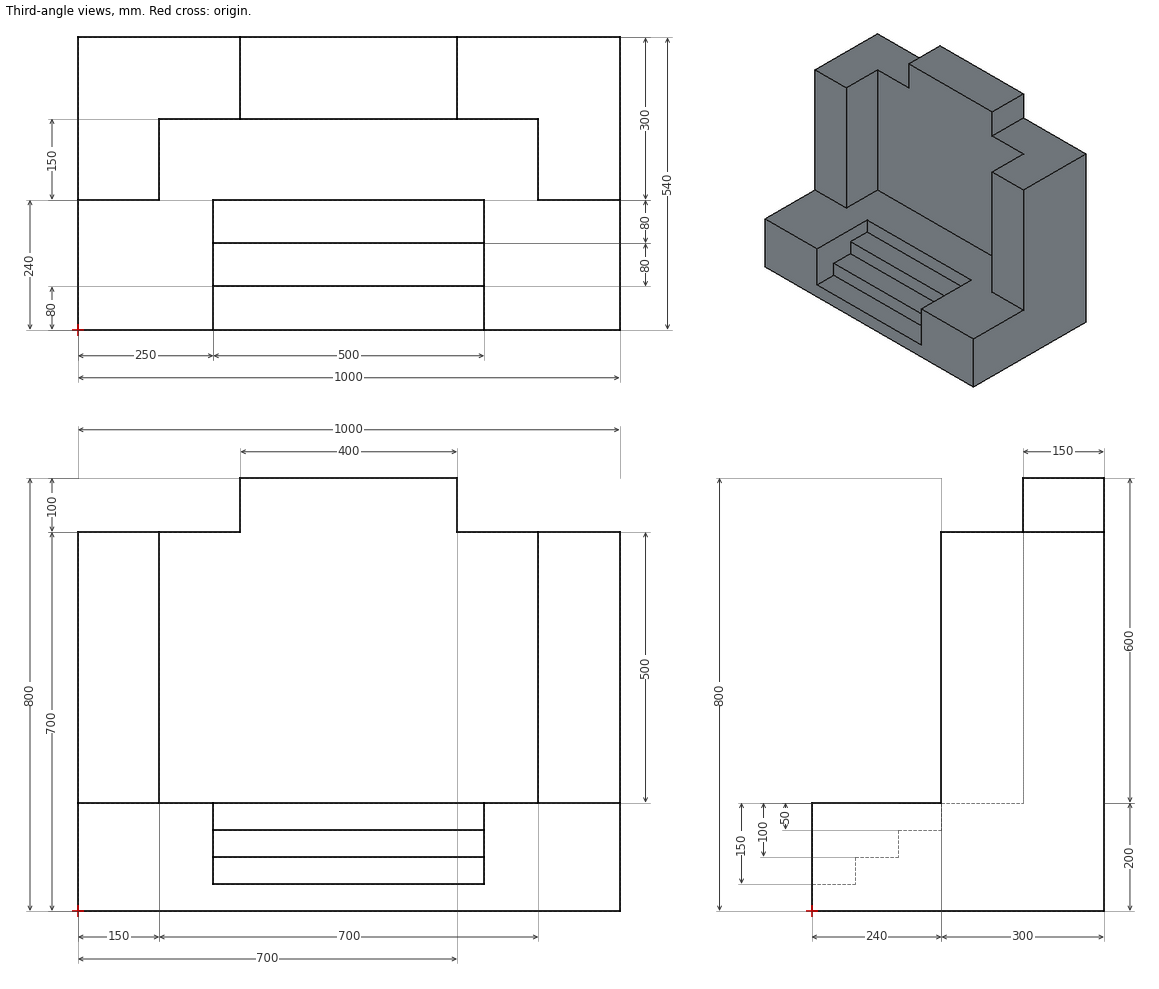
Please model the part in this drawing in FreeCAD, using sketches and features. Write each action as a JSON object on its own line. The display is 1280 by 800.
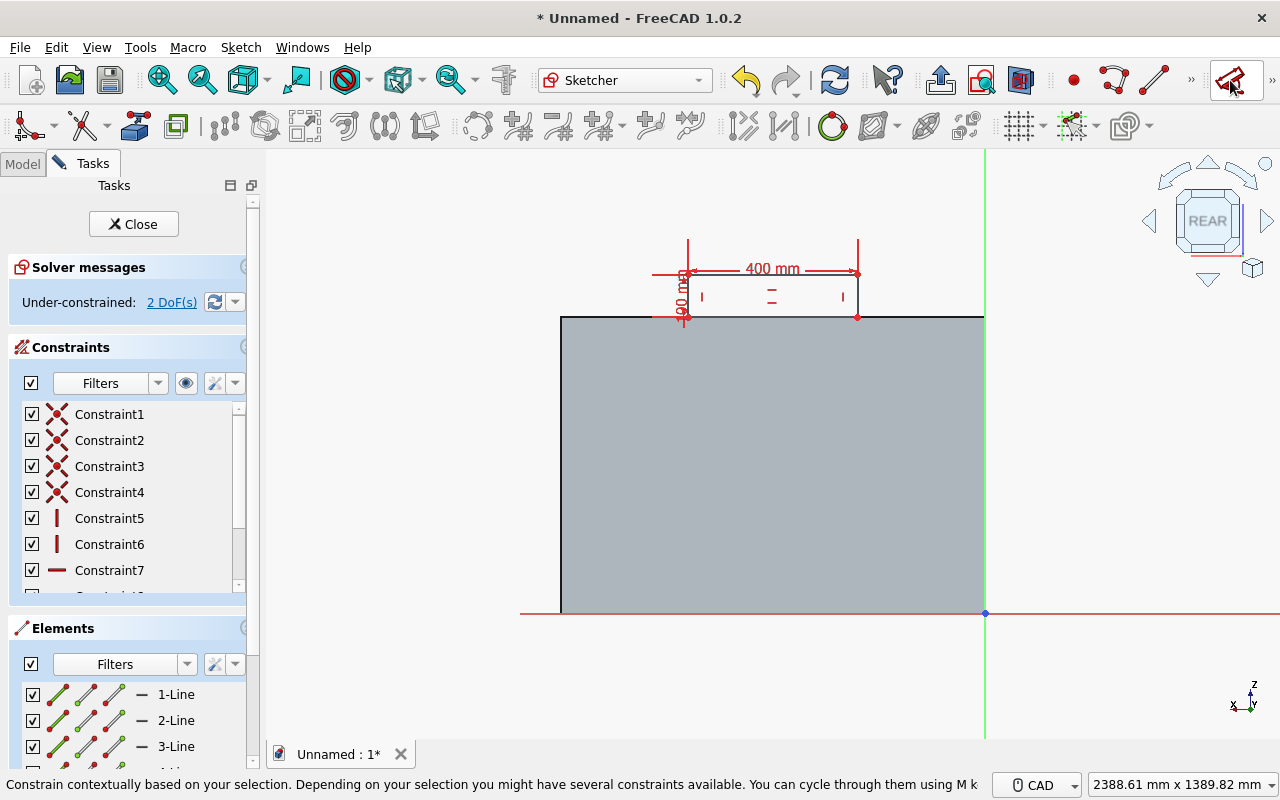
{"action": "left_click", "coordinate": [688, 275]}
{"action": "left_click", "coordinate": [837, 648]}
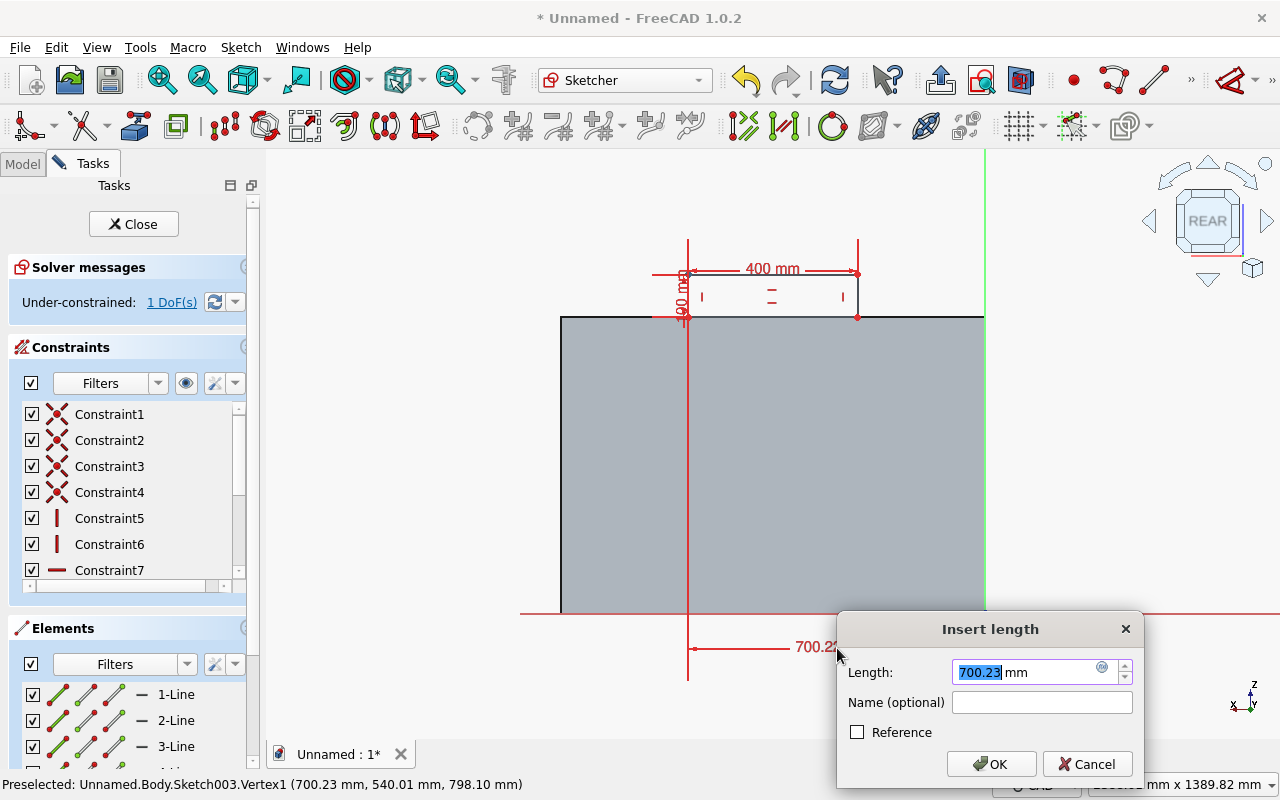
{"action": "type", "text": "700"}
{"action": "key", "text": "Return"}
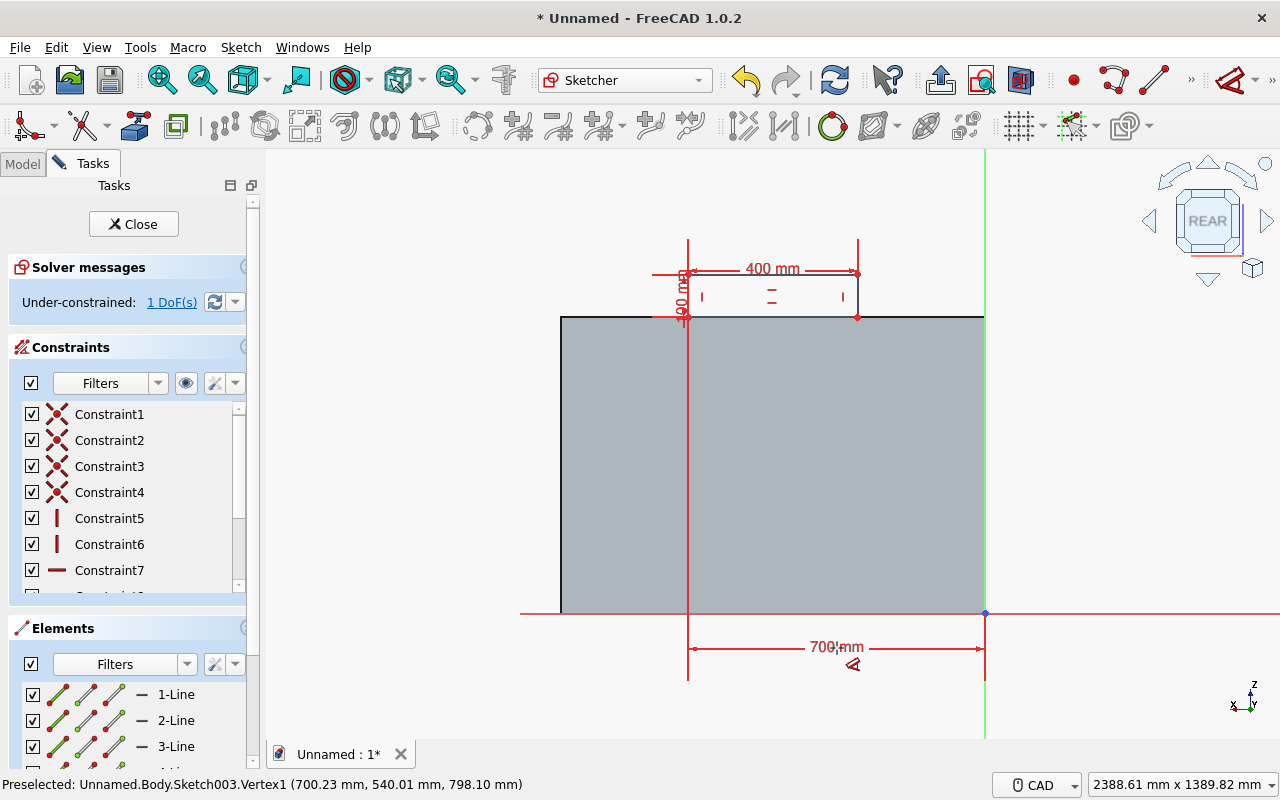
{"action": "left_click", "coordinate": [688, 275]}
{"action": "left_click", "coordinate": [1019, 444]}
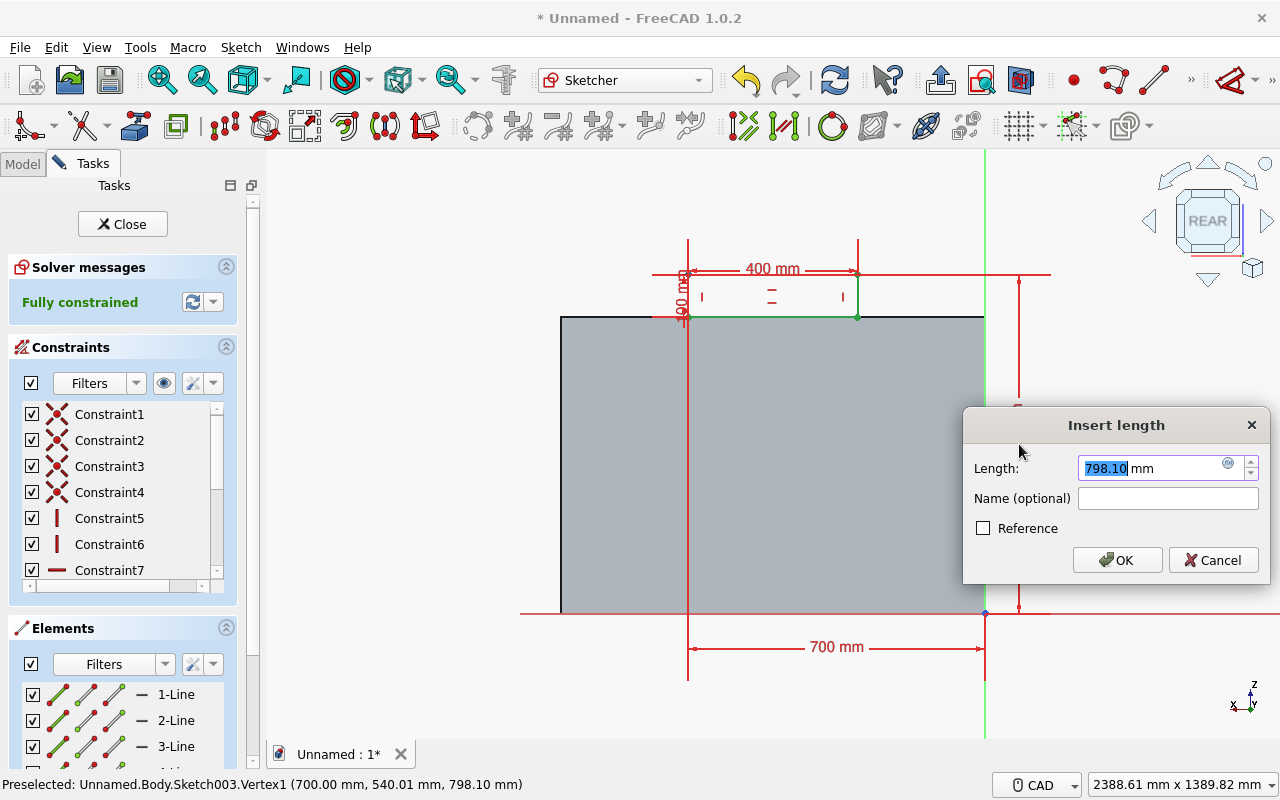
{"action": "type", "text": "800"}
{"action": "key", "text": "Return"}
{"action": "key", "text": "Escape"}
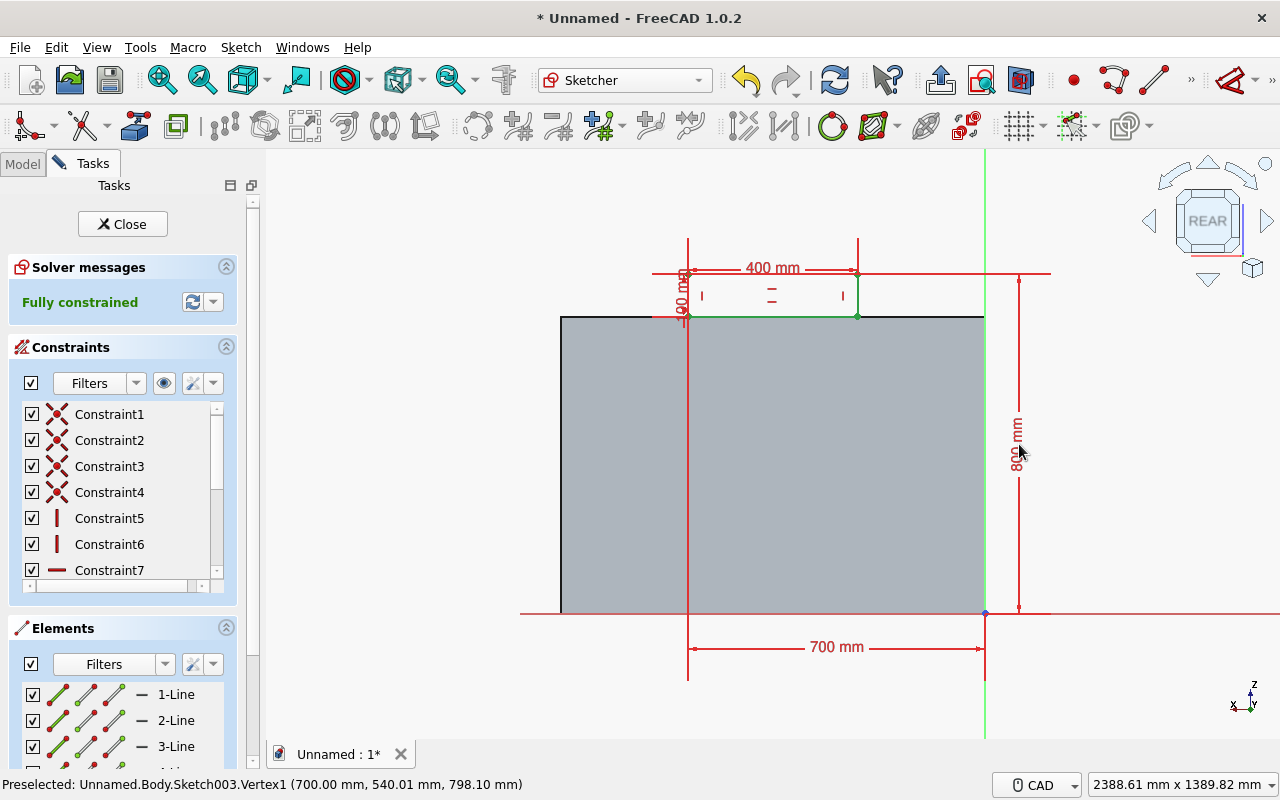
{"action": "left_click", "coordinate": [123, 224]}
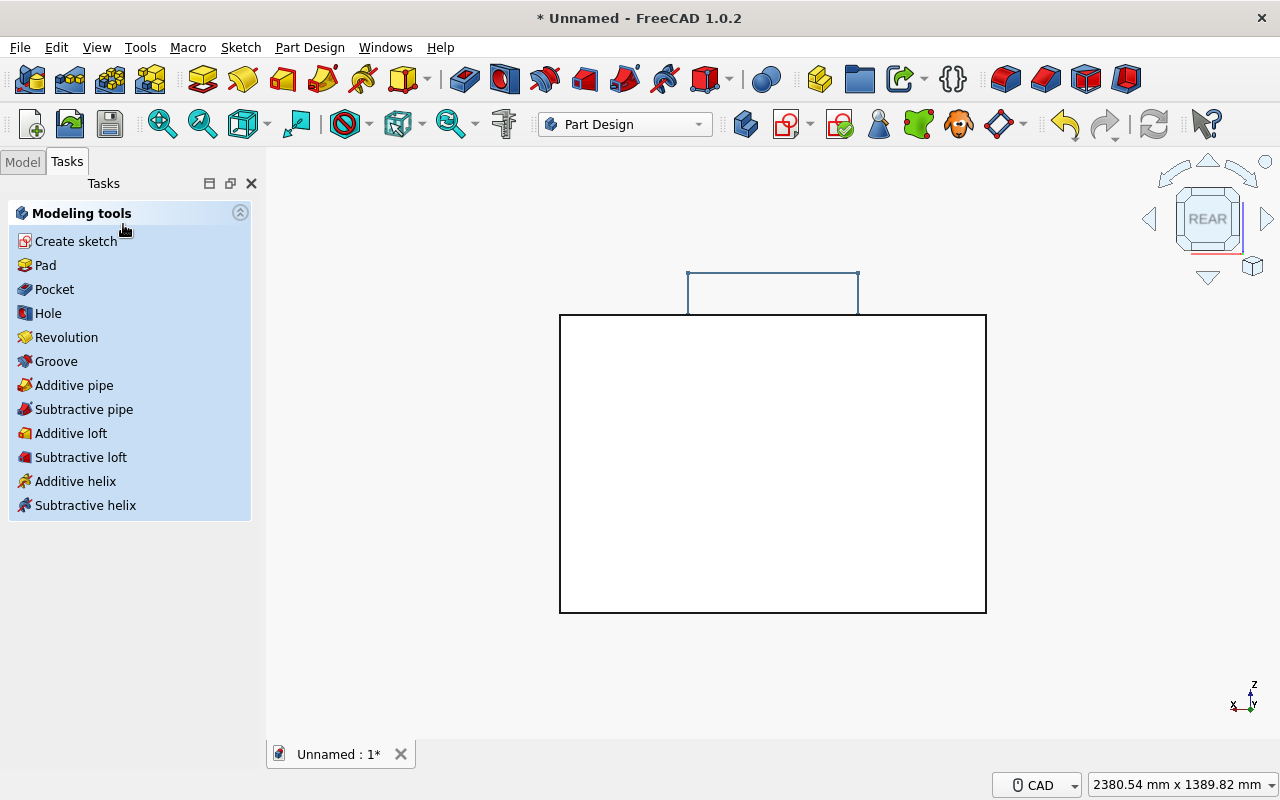
{"action": "left_click", "coordinate": [204, 80]}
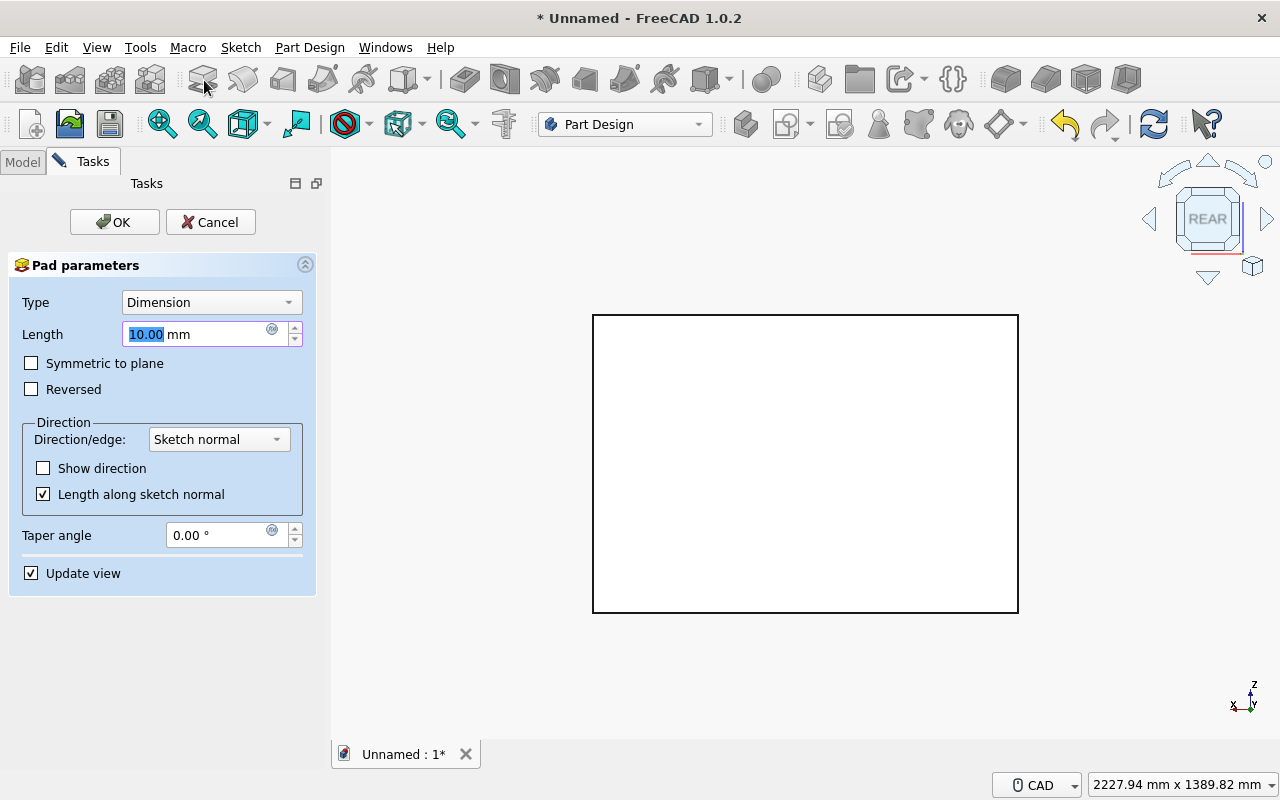
{"action": "type", "text": "150"}
{"action": "key", "text": "Tab"}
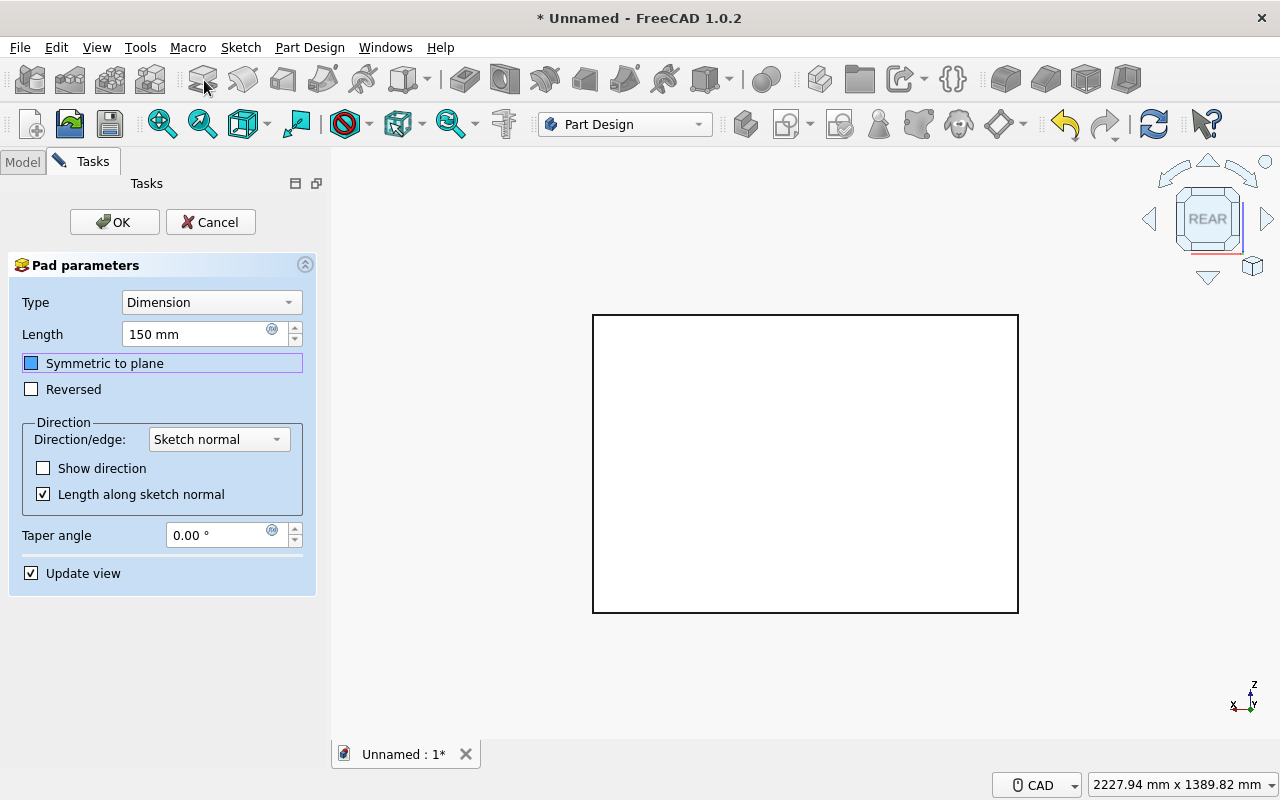
{"action": "left_click", "coordinate": [30, 389]}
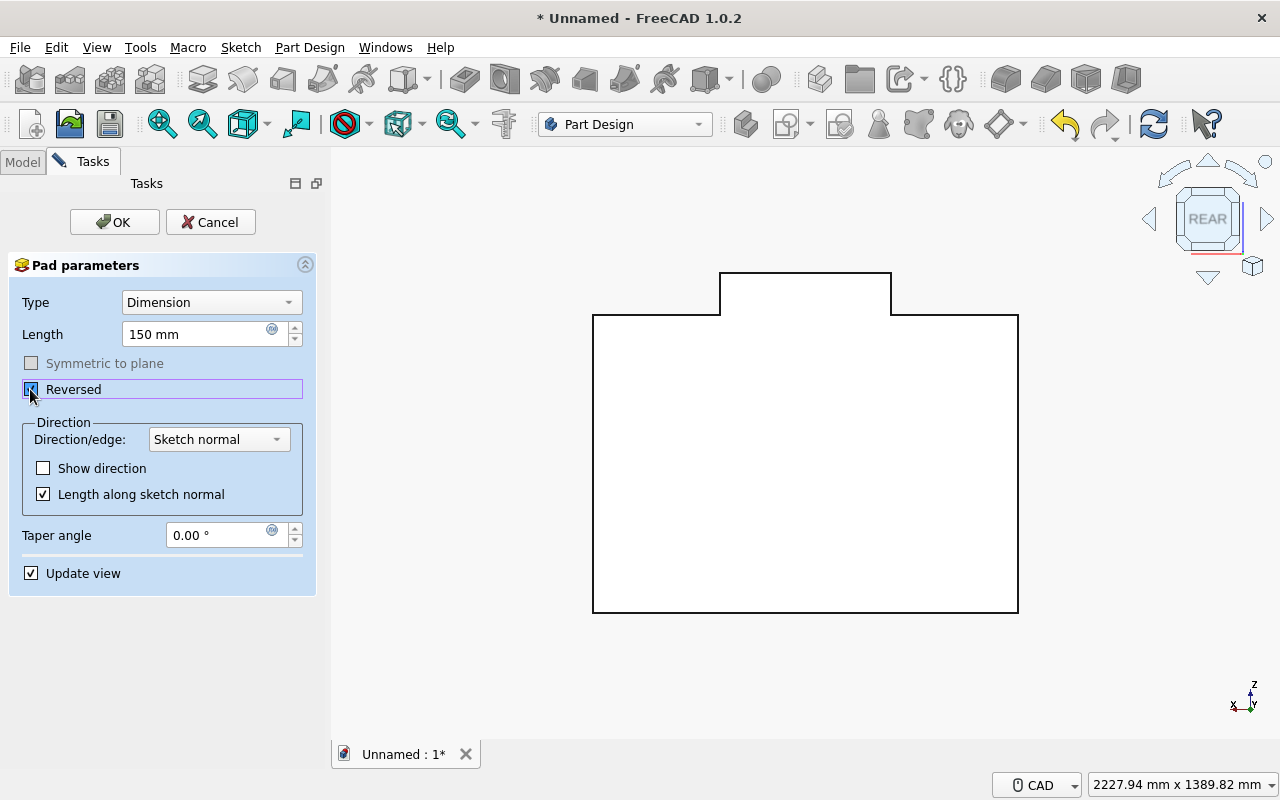
{"action": "left_click", "coordinate": [115, 222]}